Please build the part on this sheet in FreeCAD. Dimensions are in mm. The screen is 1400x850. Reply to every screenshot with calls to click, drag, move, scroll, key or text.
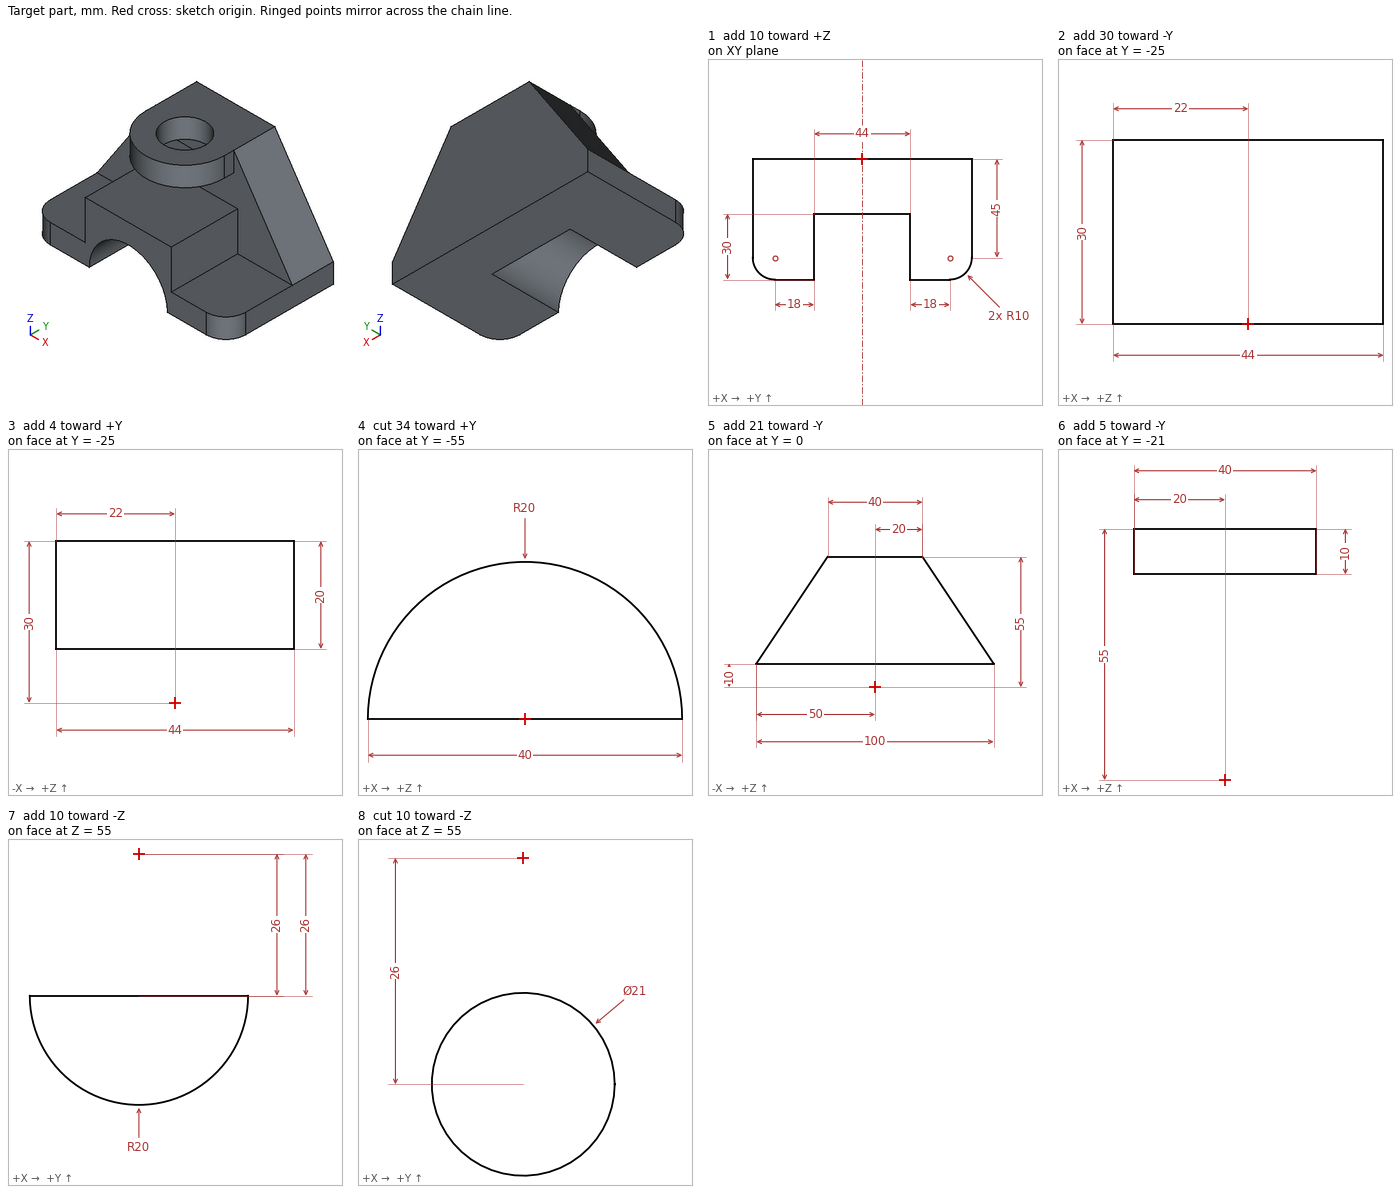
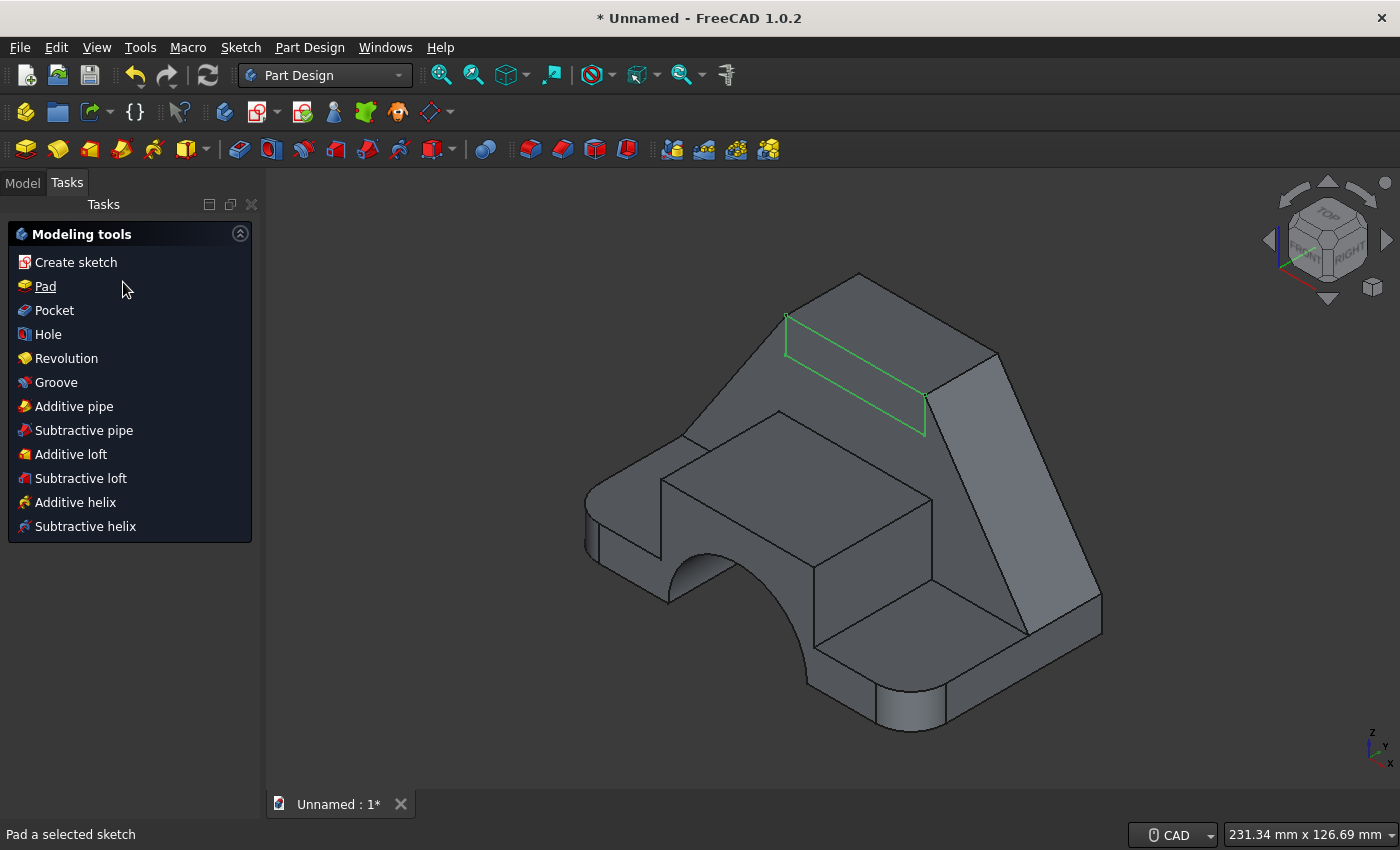
click(26, 150)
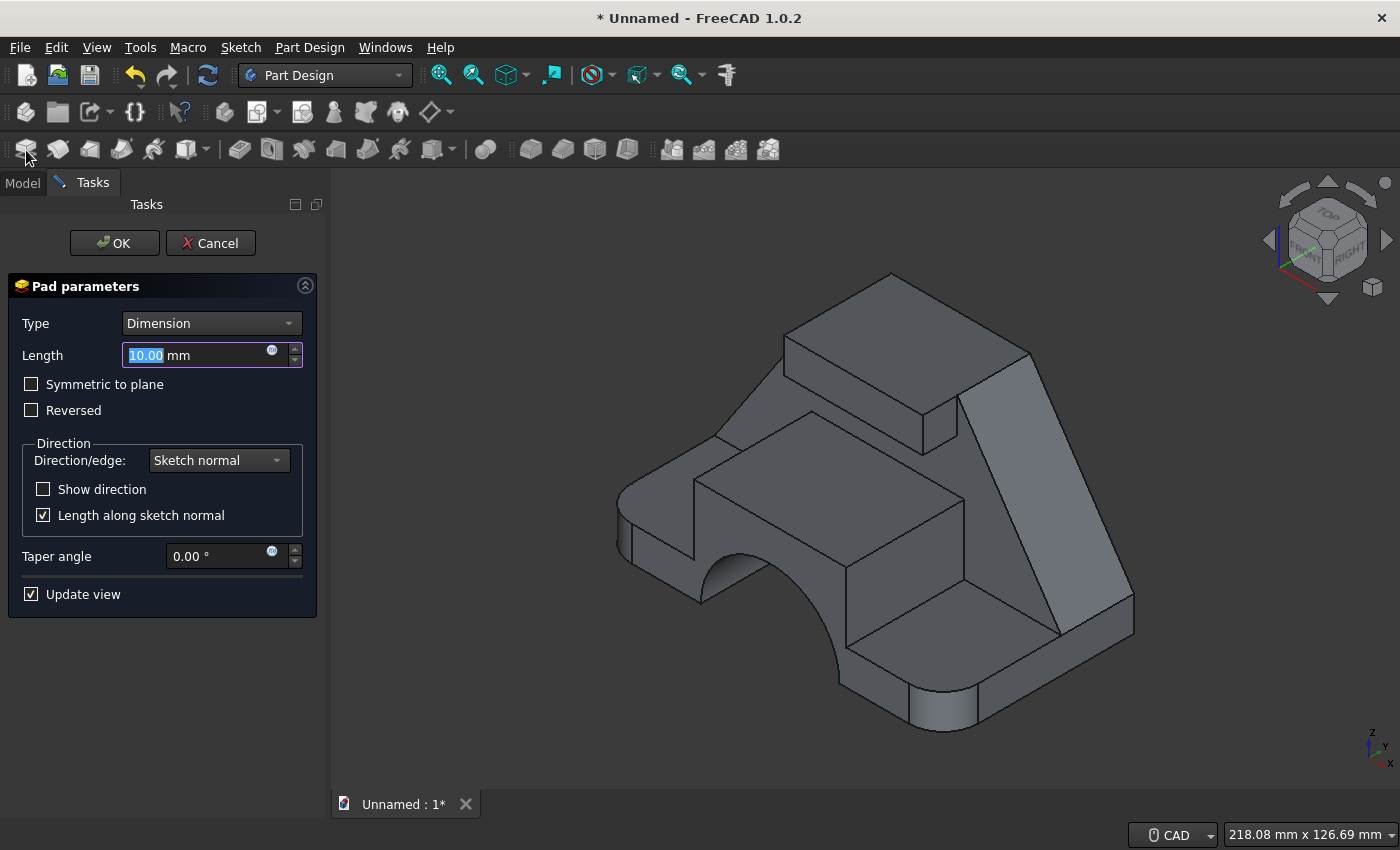
text(5)
key(Tab)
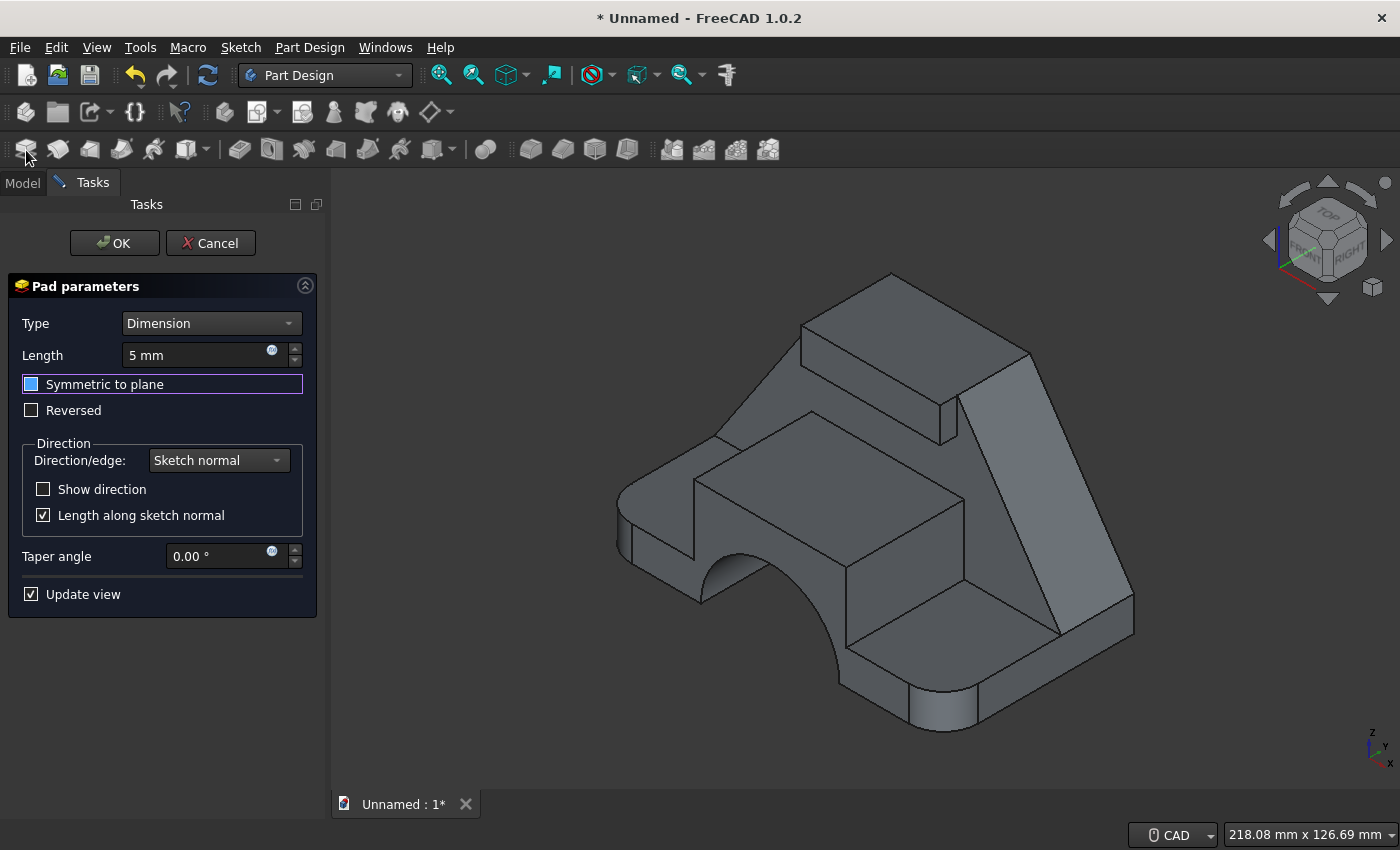
click(115, 243)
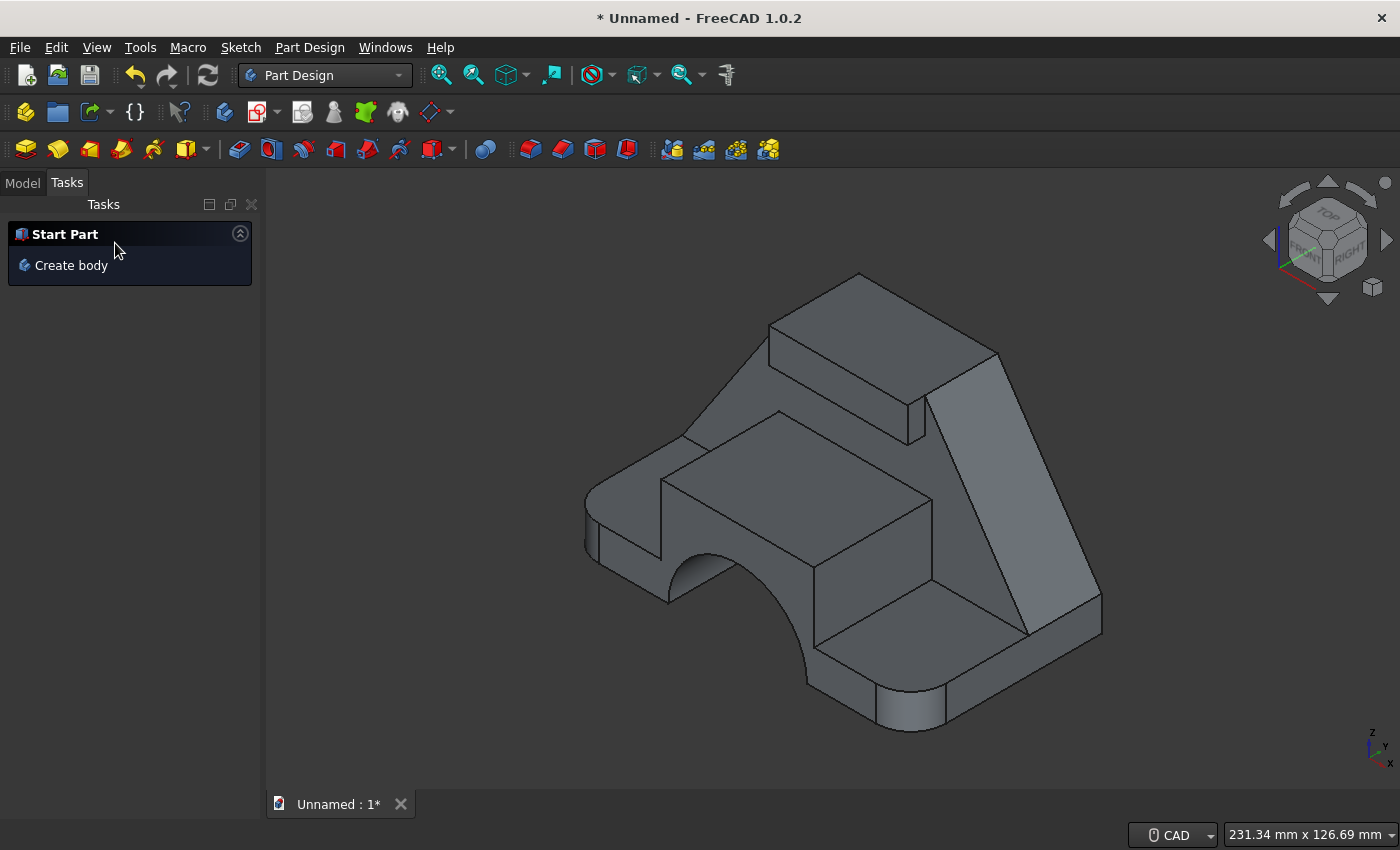
click(903, 350)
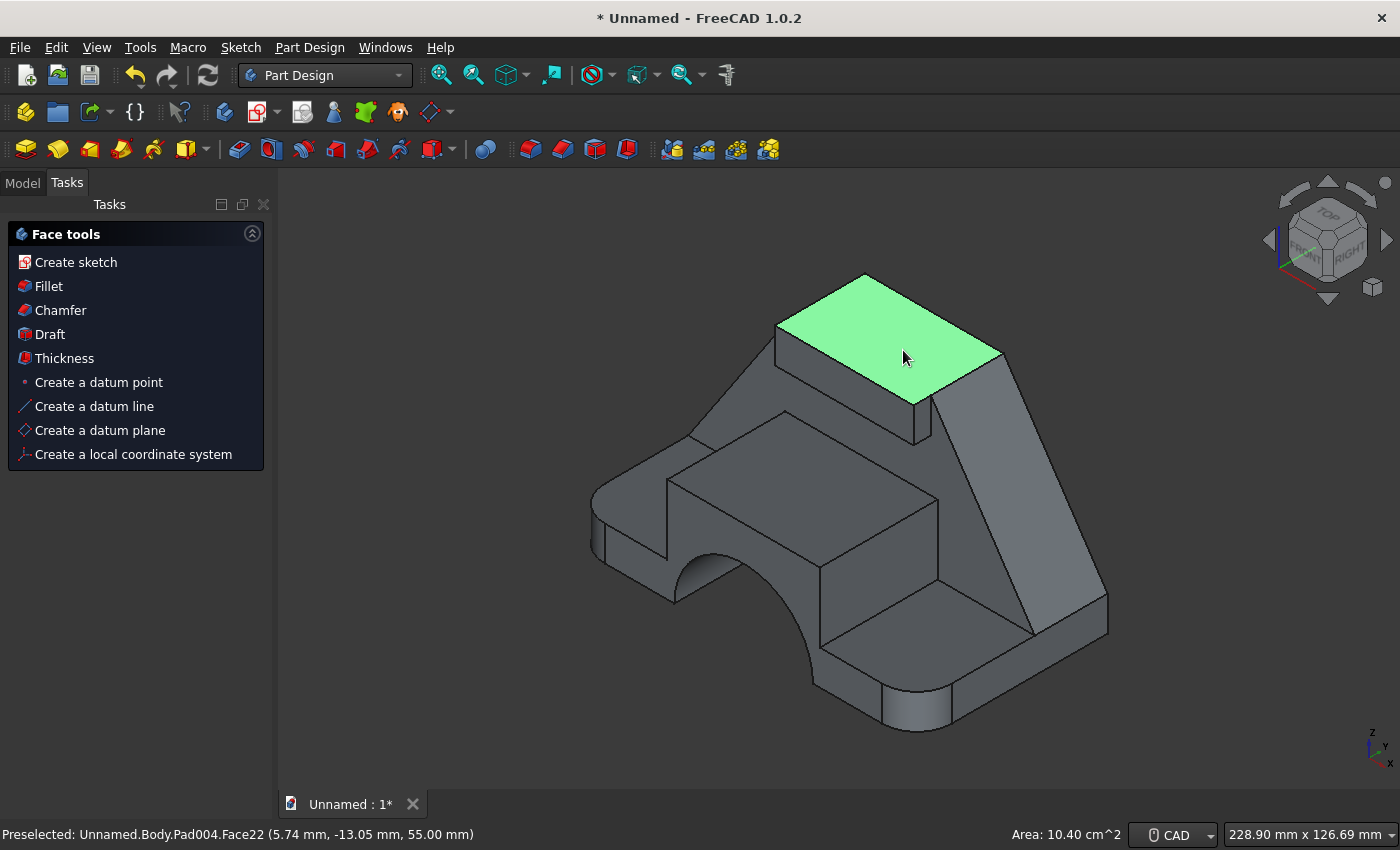
click(258, 112)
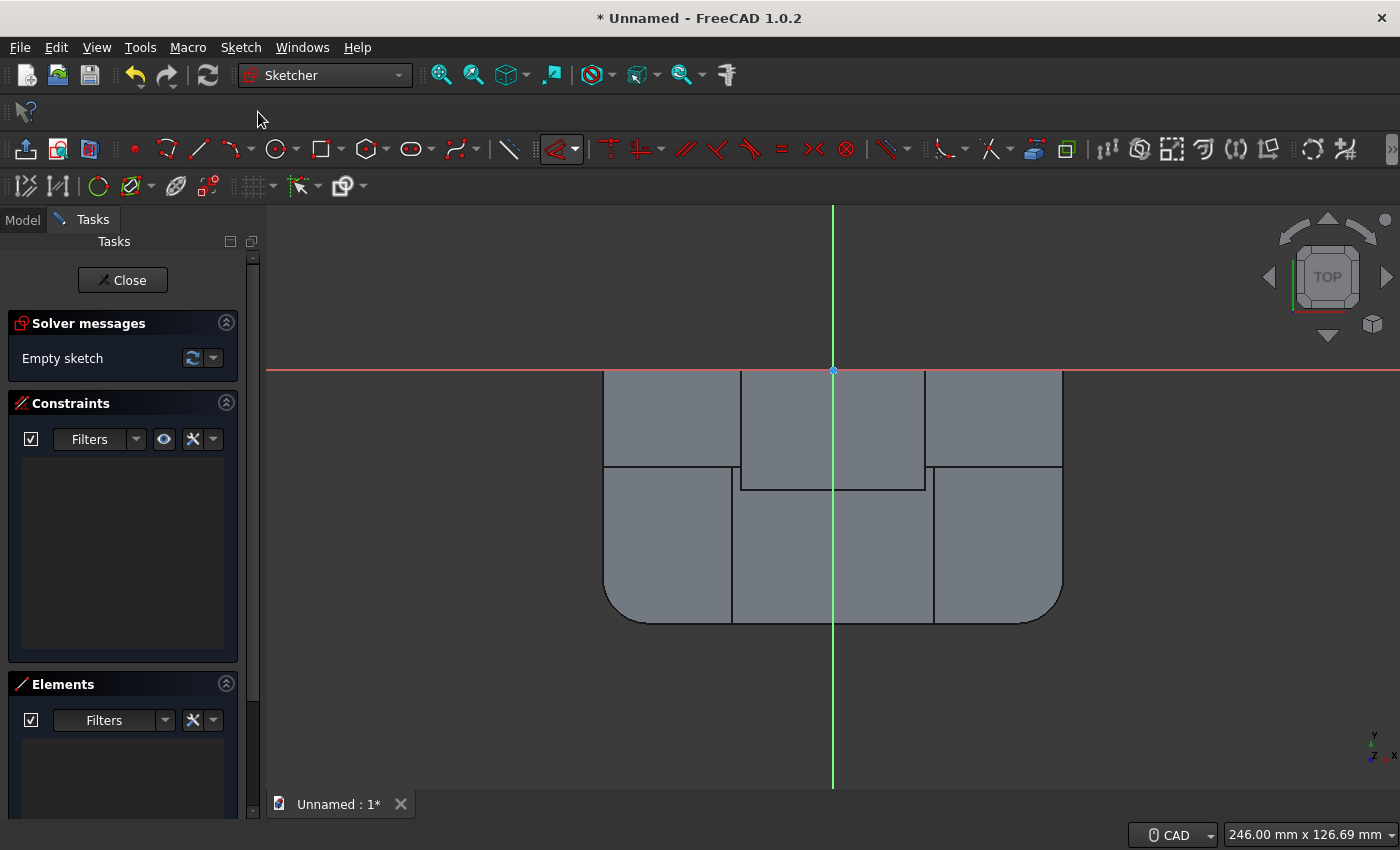
scroll(916, 451, up, 3)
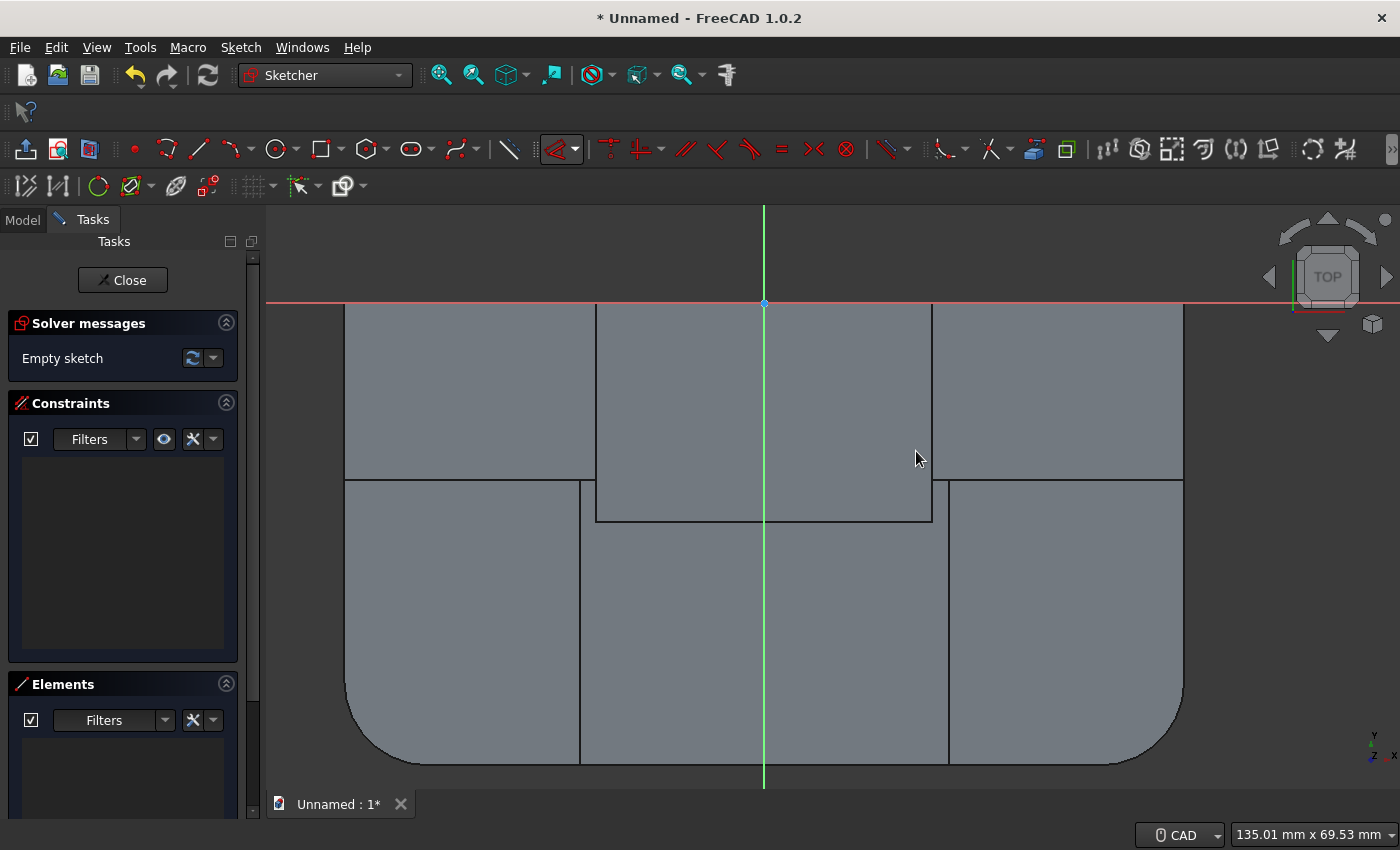
click(200, 150)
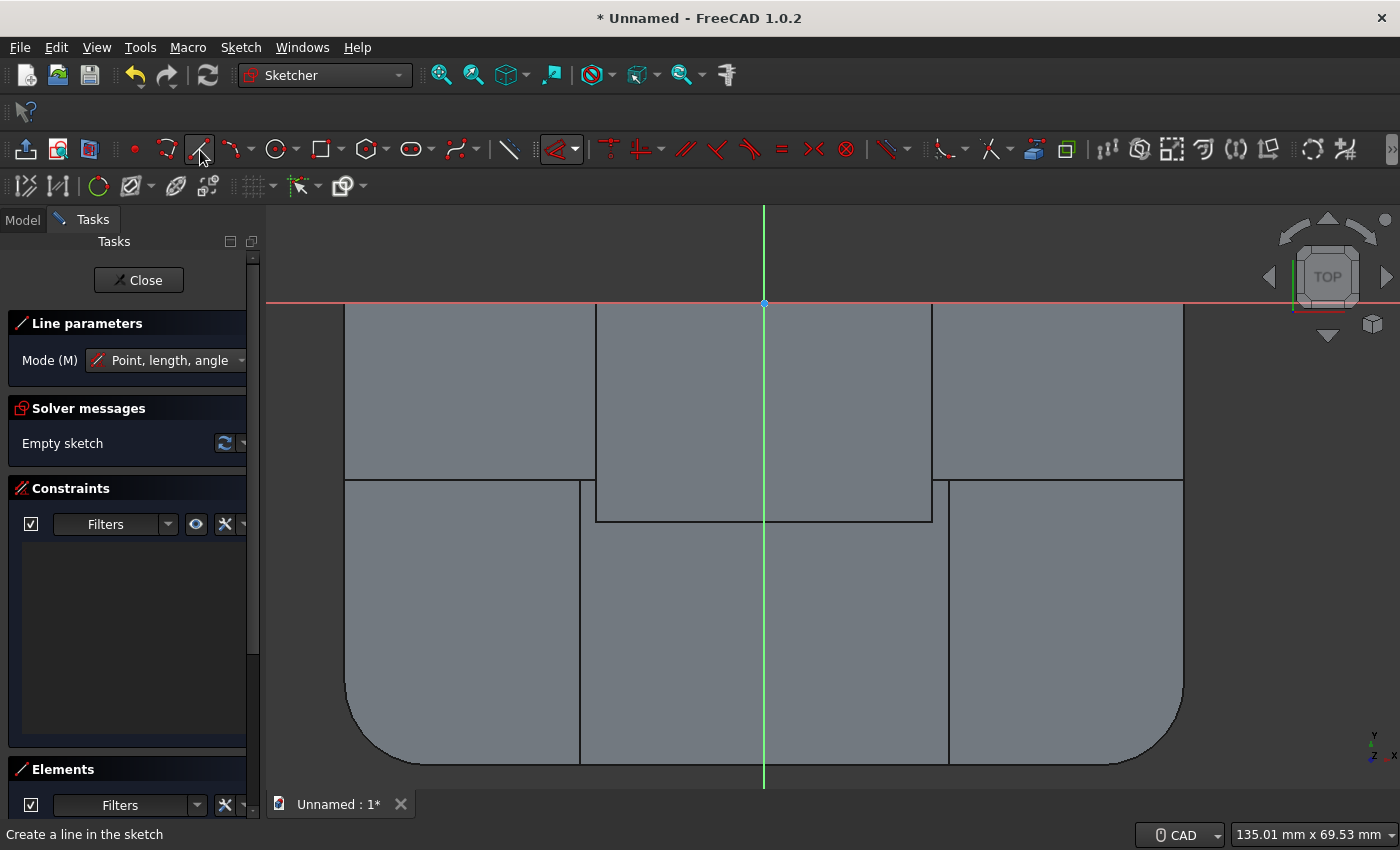
click(932, 522)
click(596, 522)